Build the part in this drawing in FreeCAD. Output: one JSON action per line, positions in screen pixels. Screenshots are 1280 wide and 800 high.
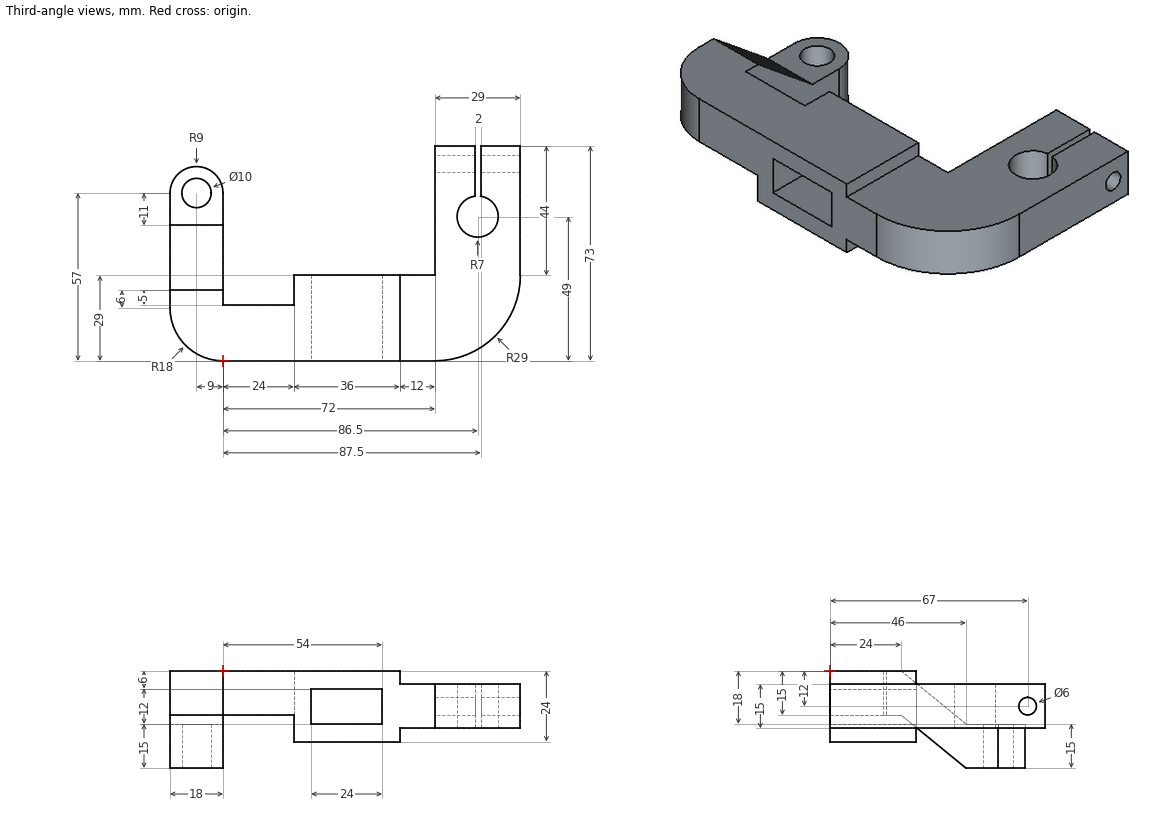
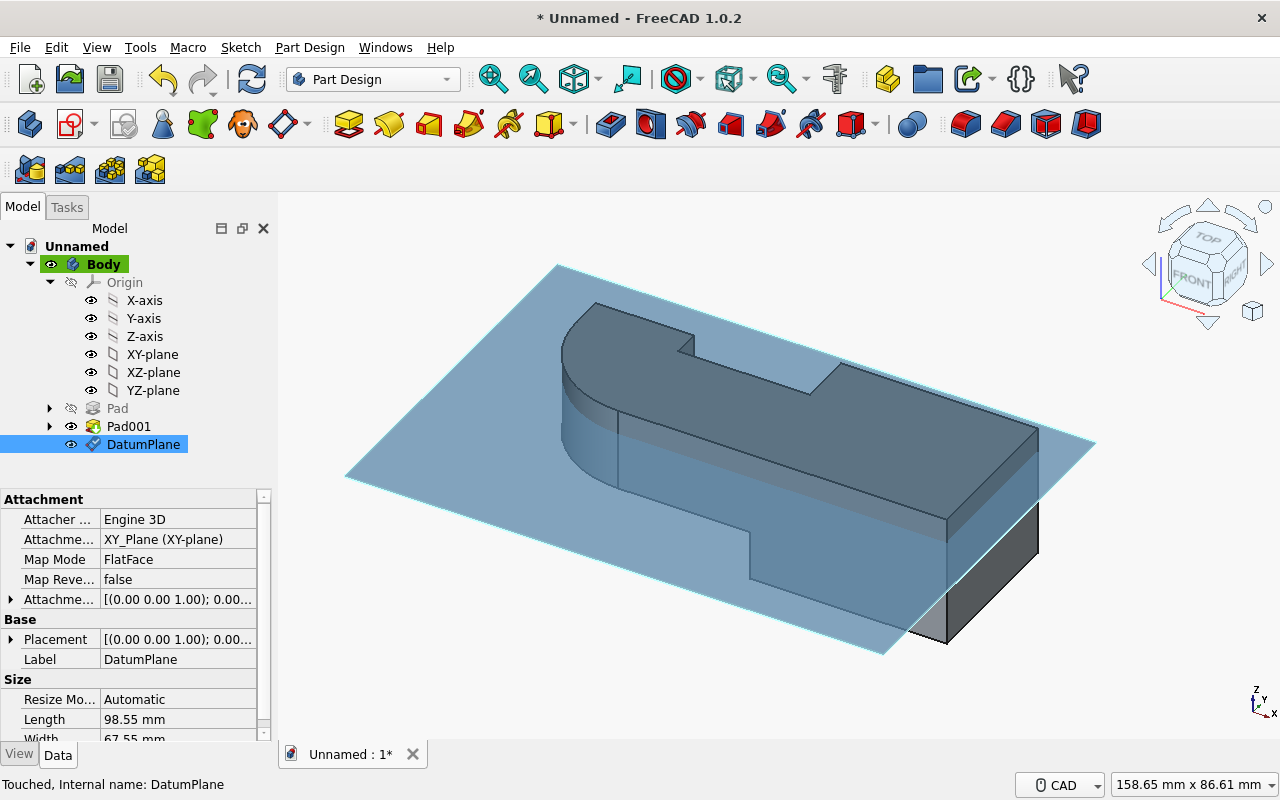
{"action": "left_click", "coordinate": [70, 124]}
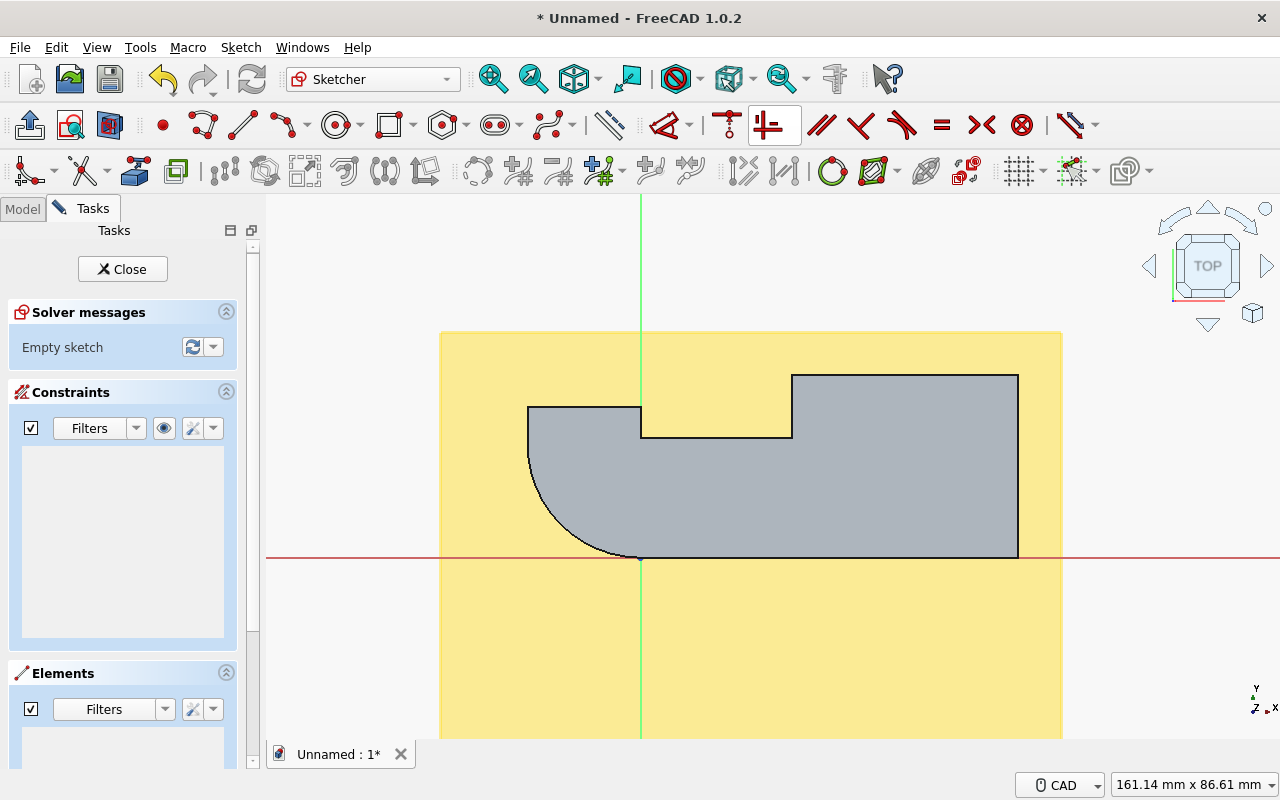
{"action": "left_click", "coordinate": [110, 126]}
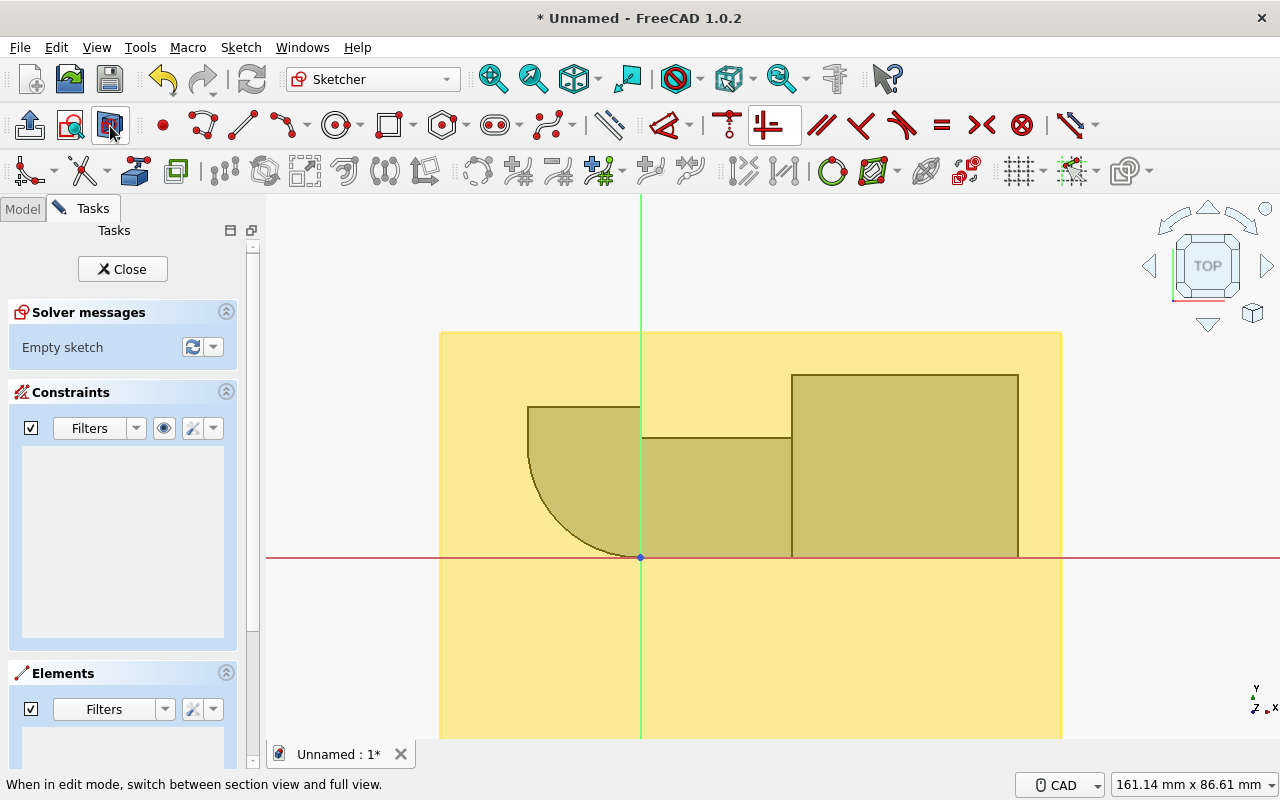
{"action": "scroll", "coordinate": [294, 711], "scroll_direction": "down", "scroll_amount": 2}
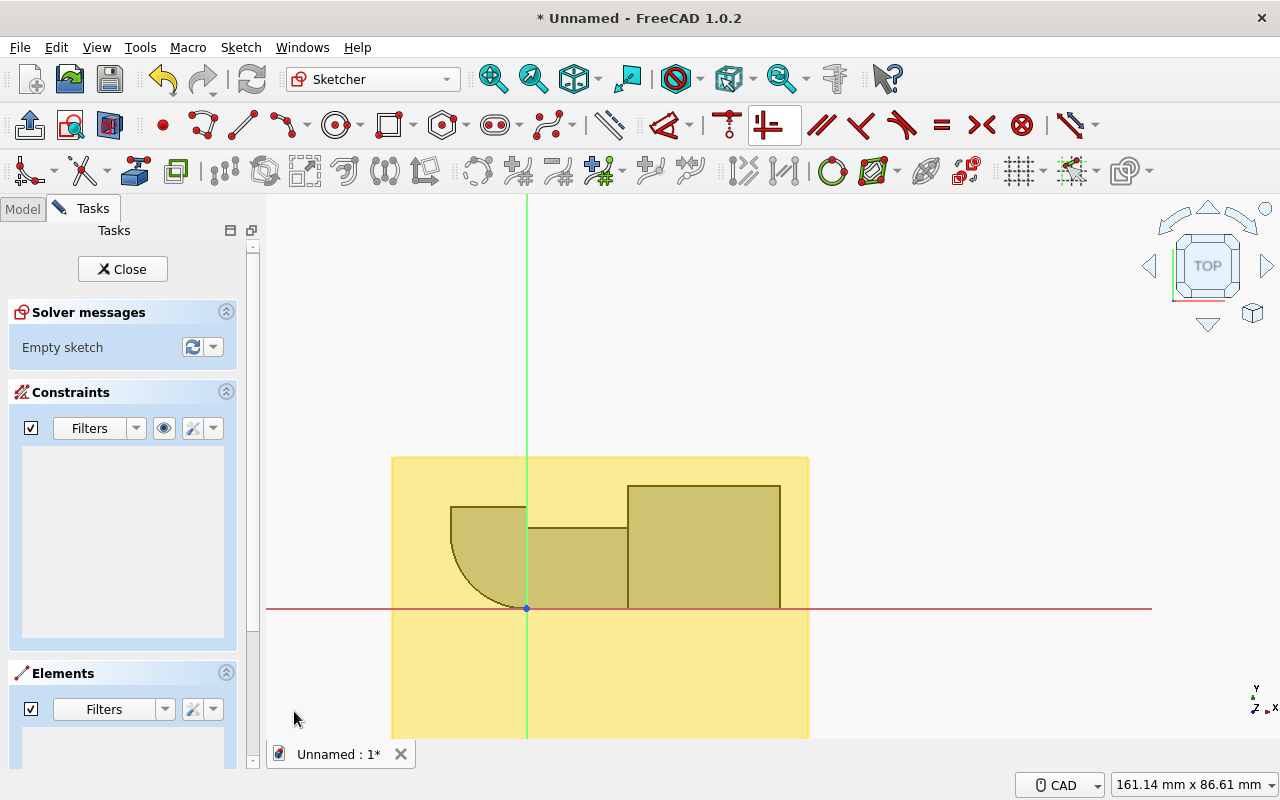
{"action": "left_click", "coordinate": [204, 126]}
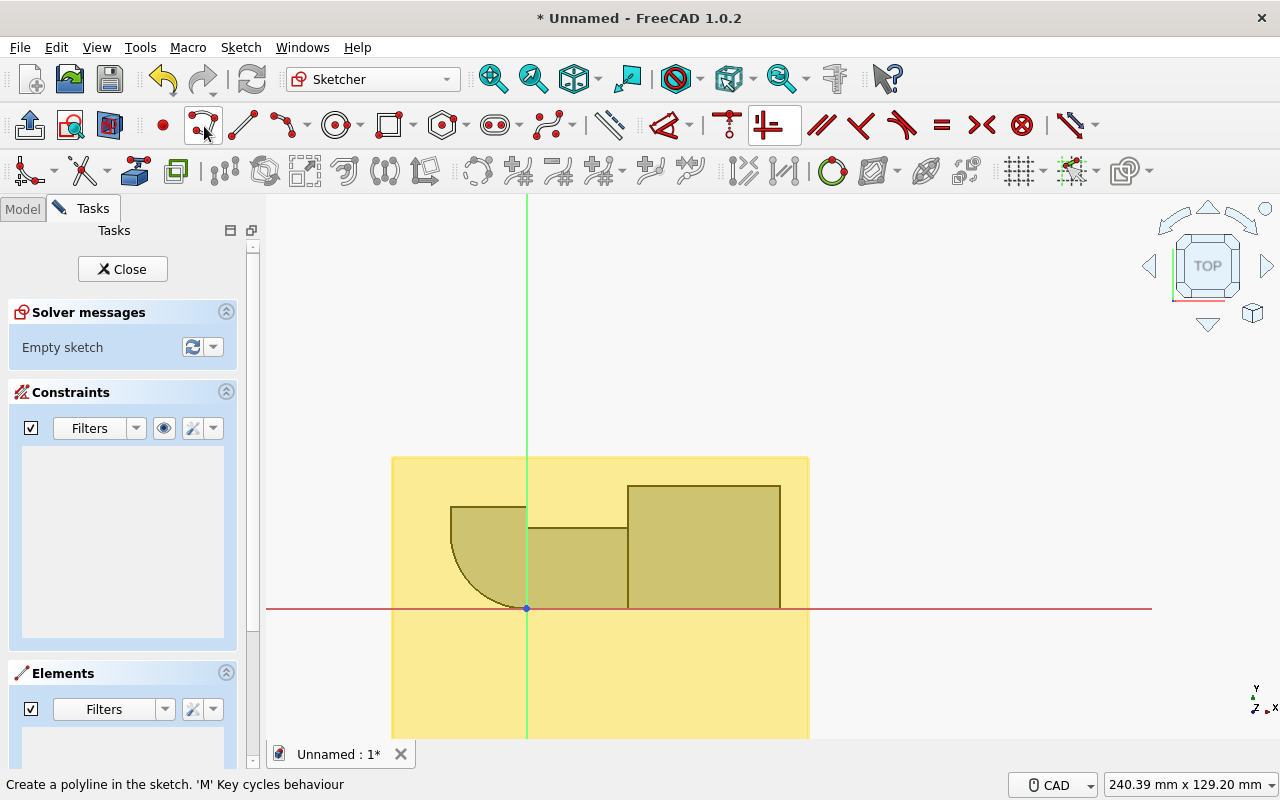
{"action": "left_click", "coordinate": [953, 486]}
{"action": "left_click", "coordinate": [953, 301]}
{"action": "left_click", "coordinate": [830, 301]}
{"action": "left_click", "coordinate": [830, 486]}
{"action": "left_click", "coordinate": [780, 486]}
{"action": "left_click", "coordinate": [780, 609]}
{"action": "left_click", "coordinate": [830, 600]}
{"action": "right_click", "coordinate": [830, 600]}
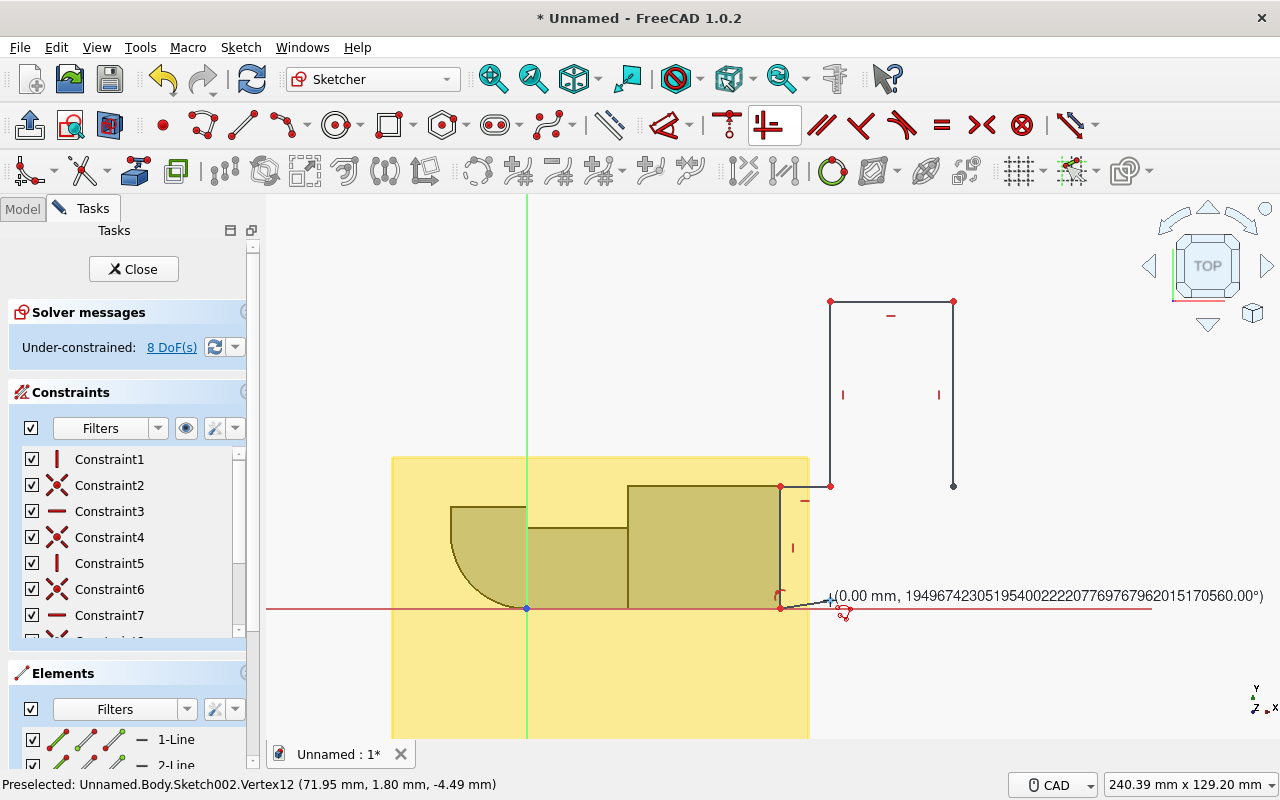
{"action": "left_click", "coordinate": [284, 126]}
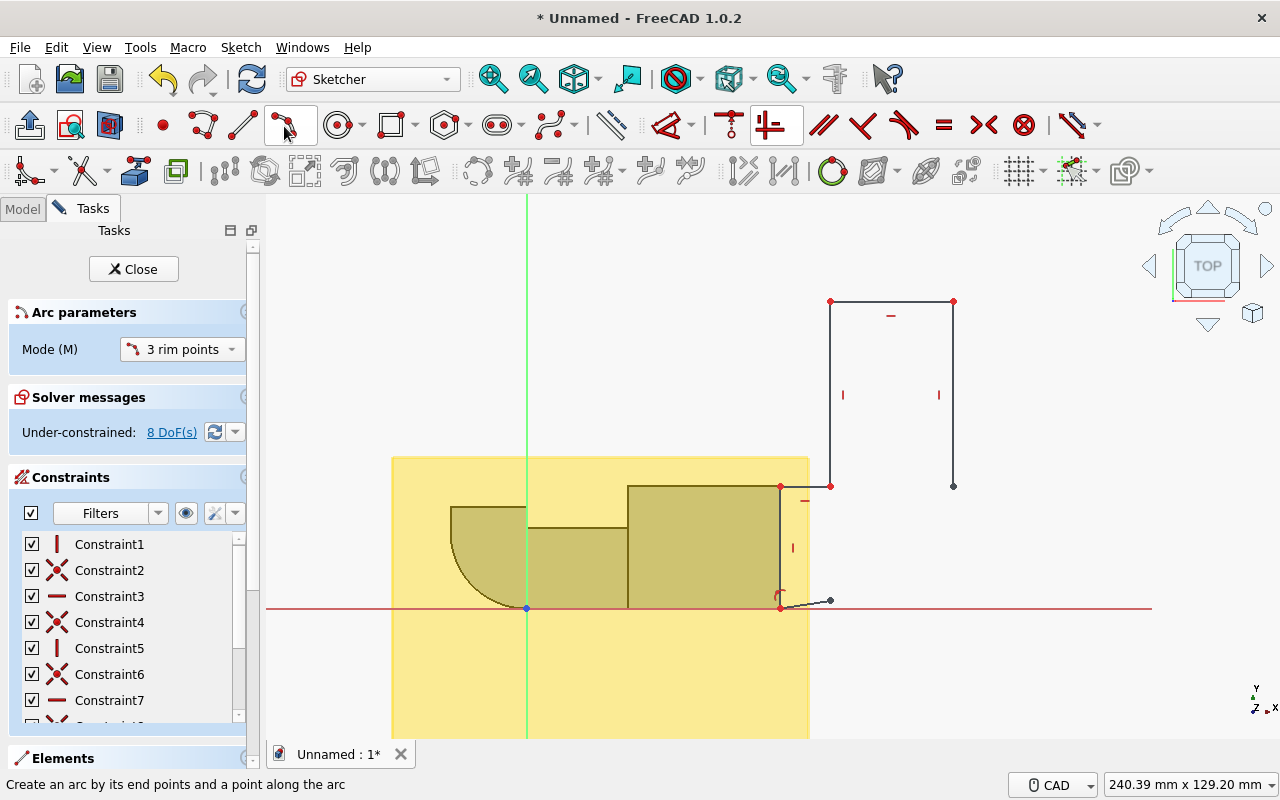
{"action": "left_click", "coordinate": [830, 601]}
{"action": "left_click", "coordinate": [953, 487]}
{"action": "left_click", "coordinate": [917, 573]}
{"action": "key", "text": "Escape"}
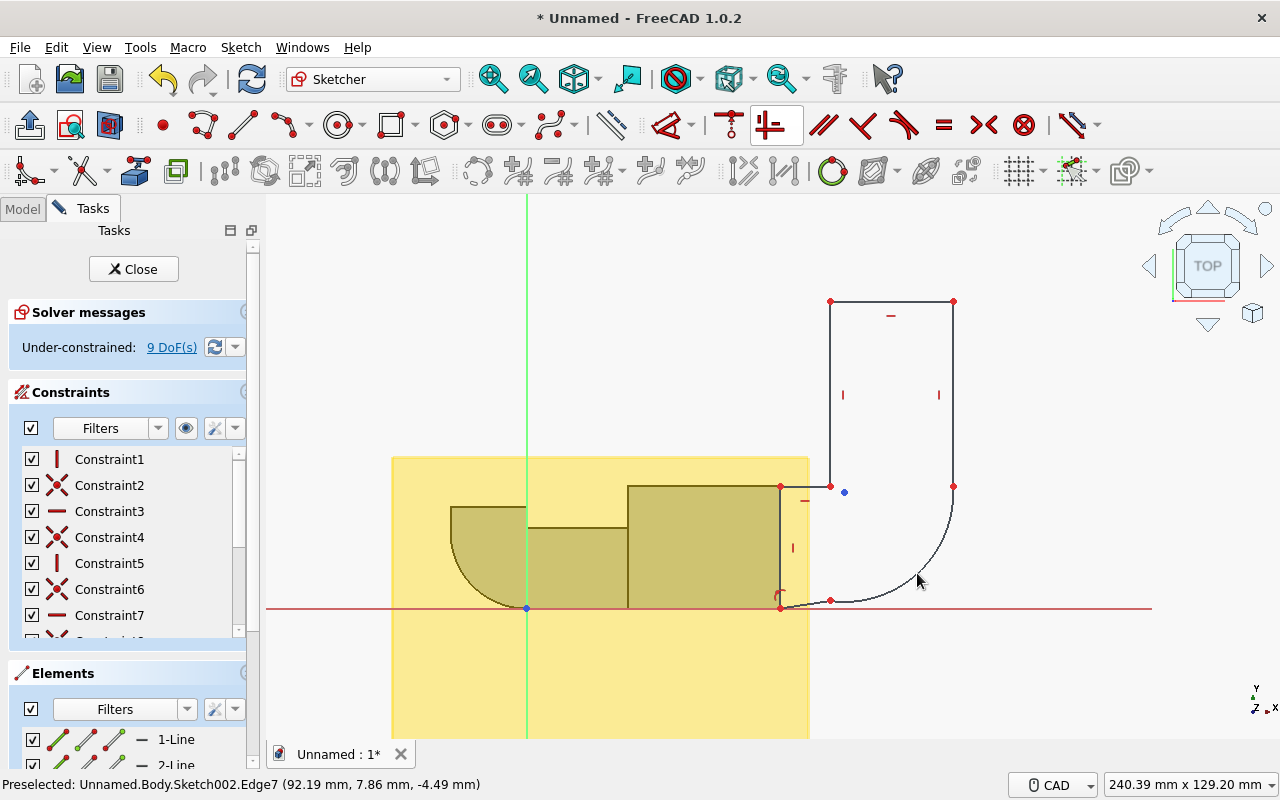
{"action": "left_click", "coordinate": [953, 431]}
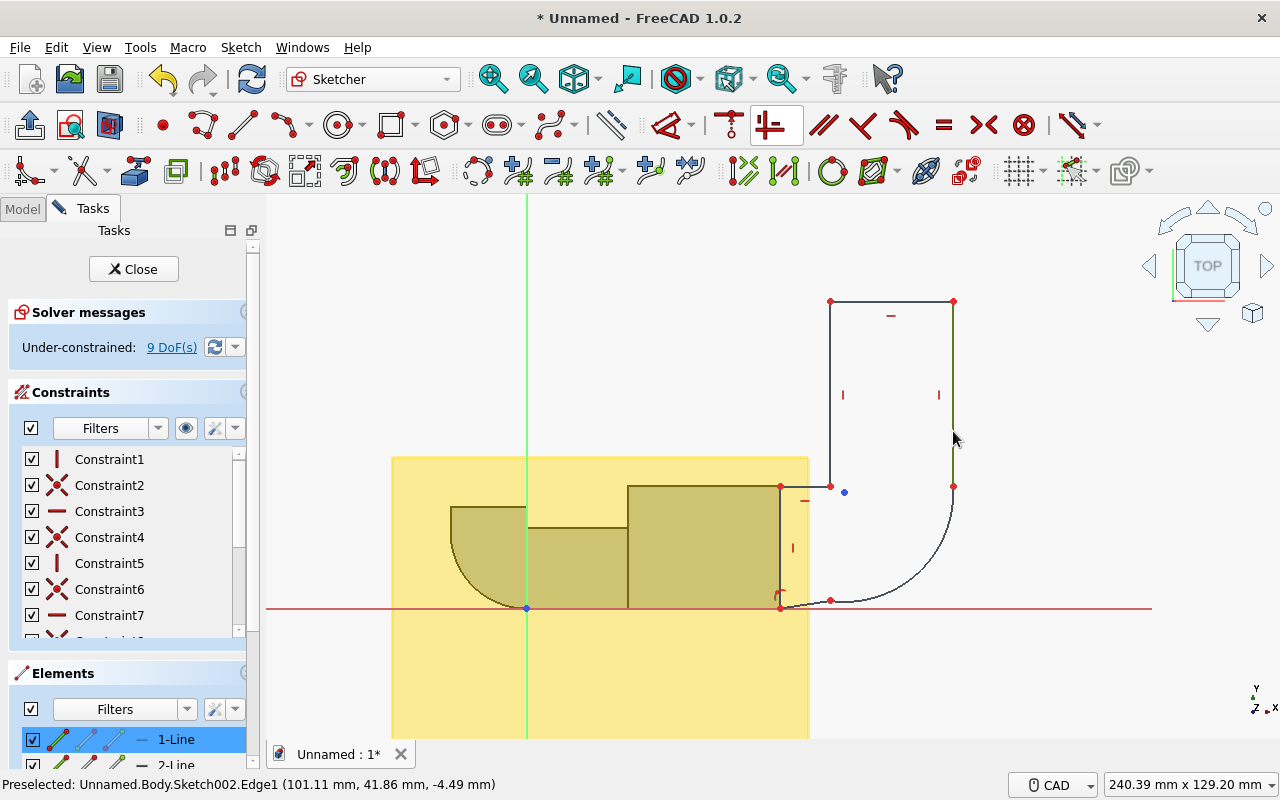
{"action": "left_click", "coordinate": [886, 593]}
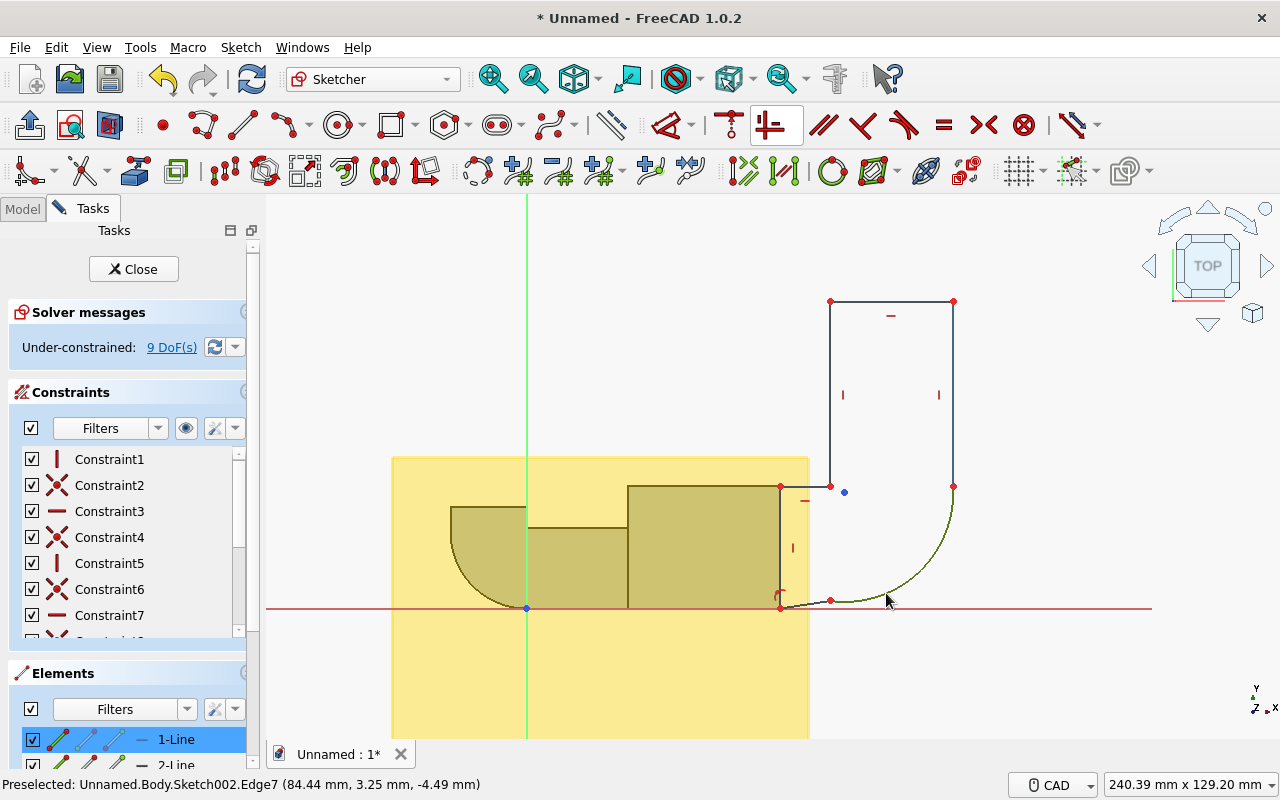
{"action": "left_click", "coordinate": [904, 126]}